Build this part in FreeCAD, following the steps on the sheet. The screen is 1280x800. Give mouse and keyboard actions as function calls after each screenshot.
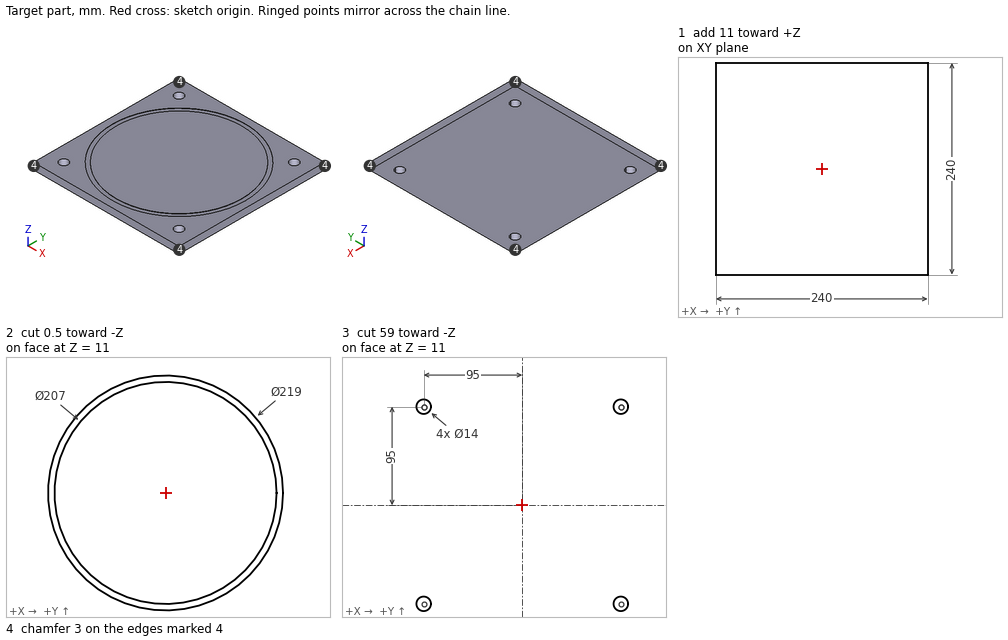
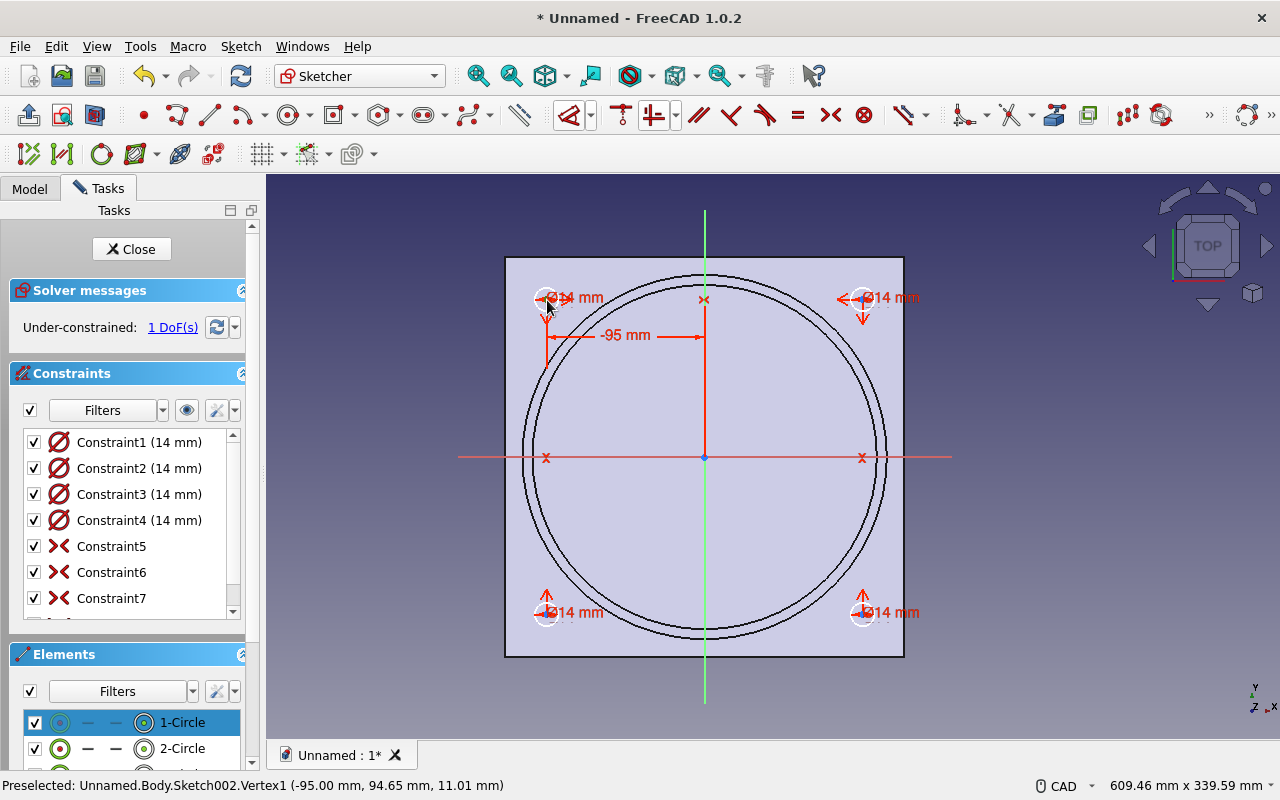
key(i)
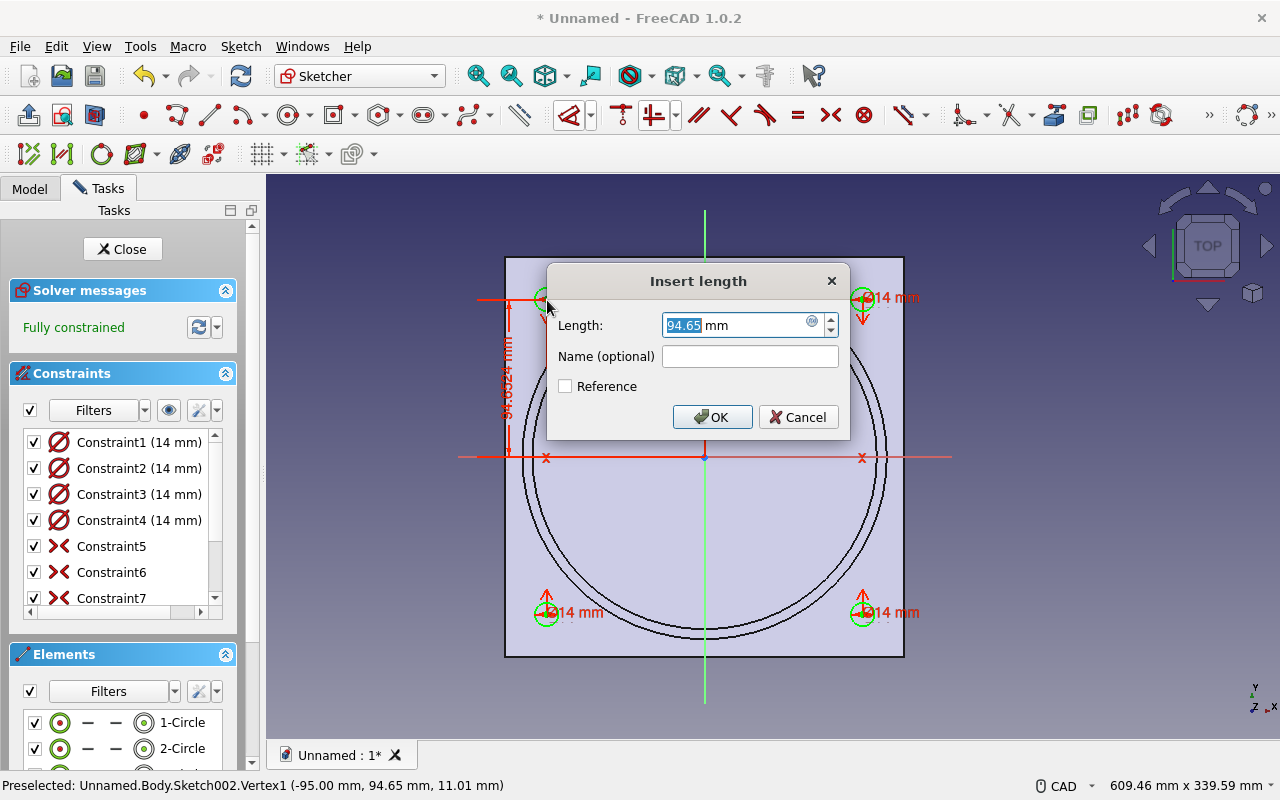
text(95)
key(Return)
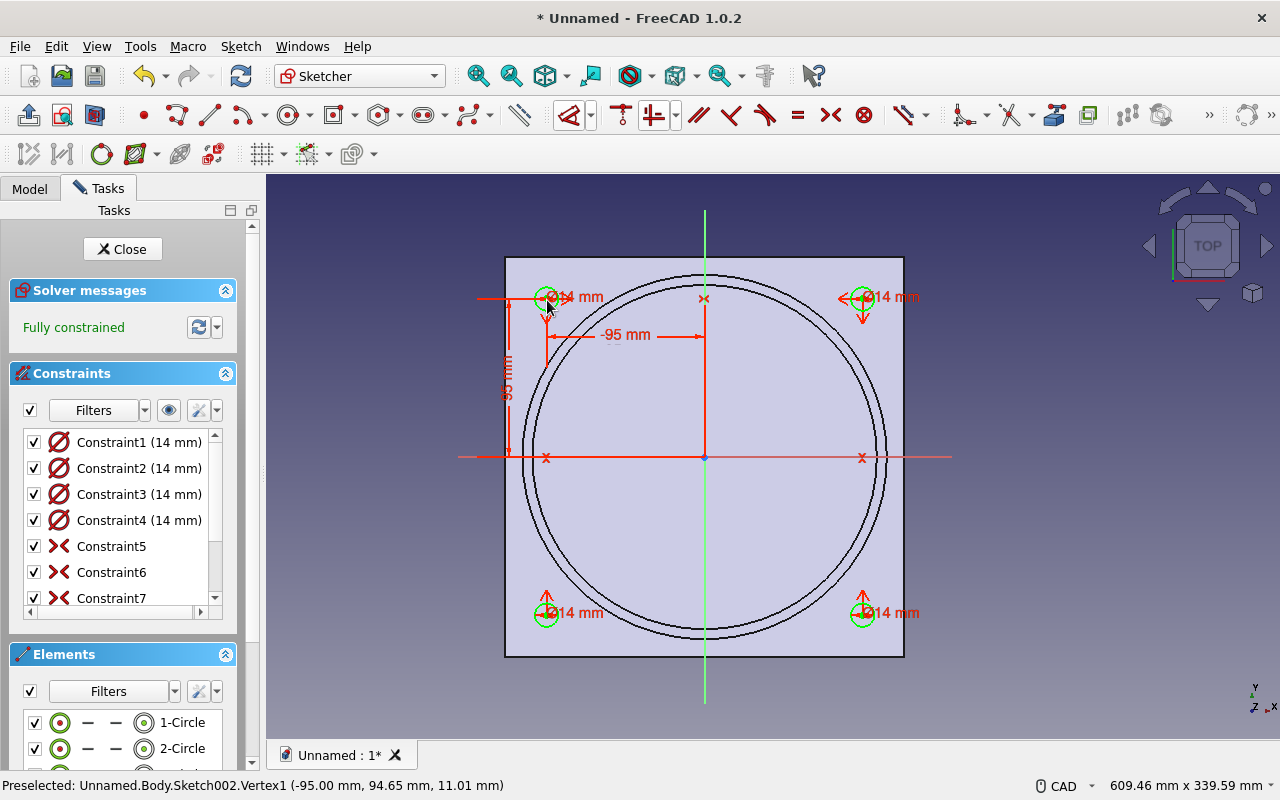
click(123, 249)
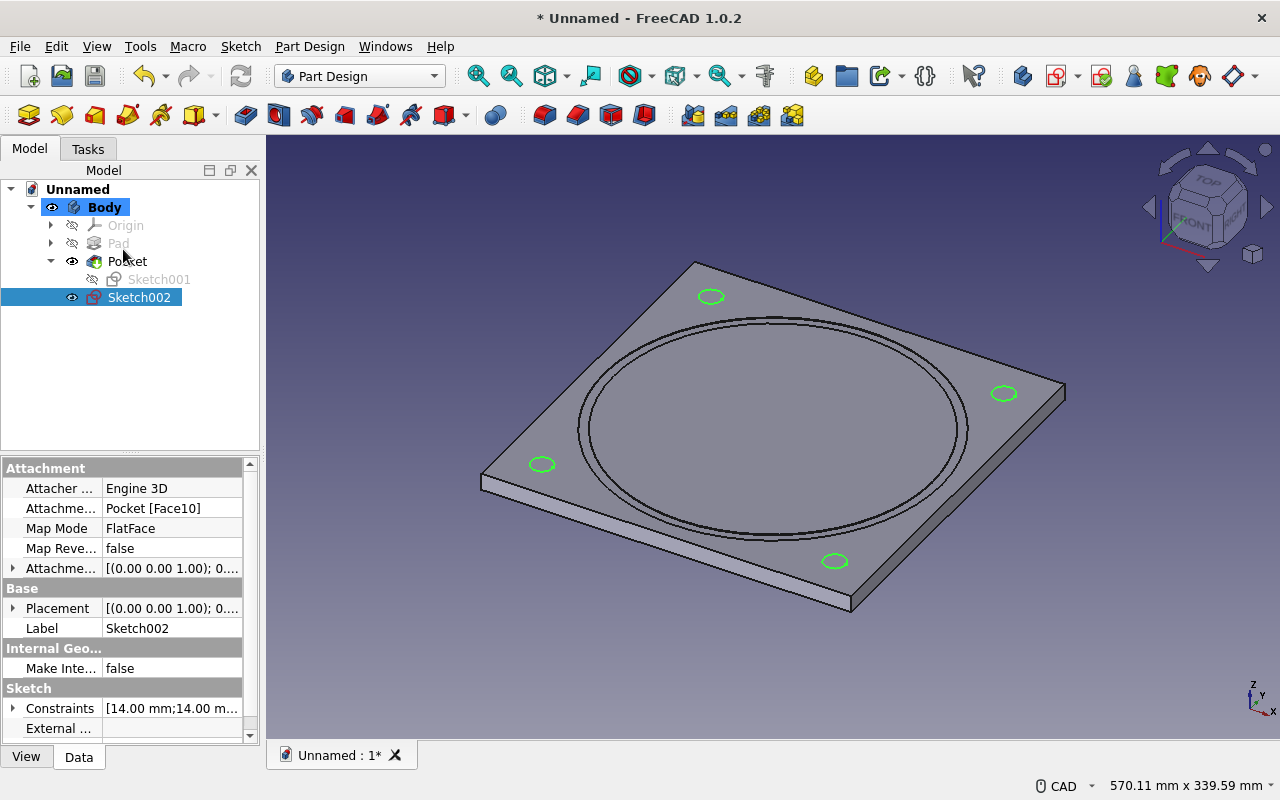
click(246, 116)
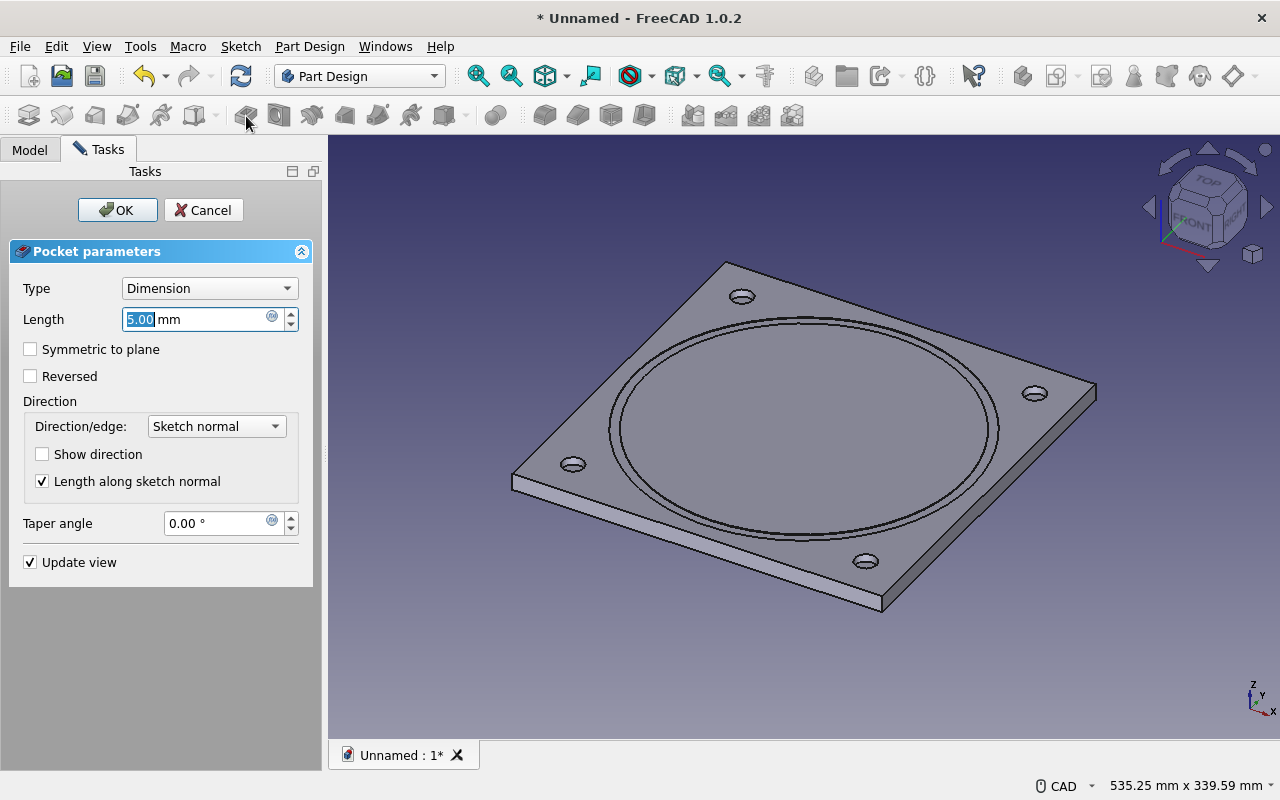
text(59)
key(Tab)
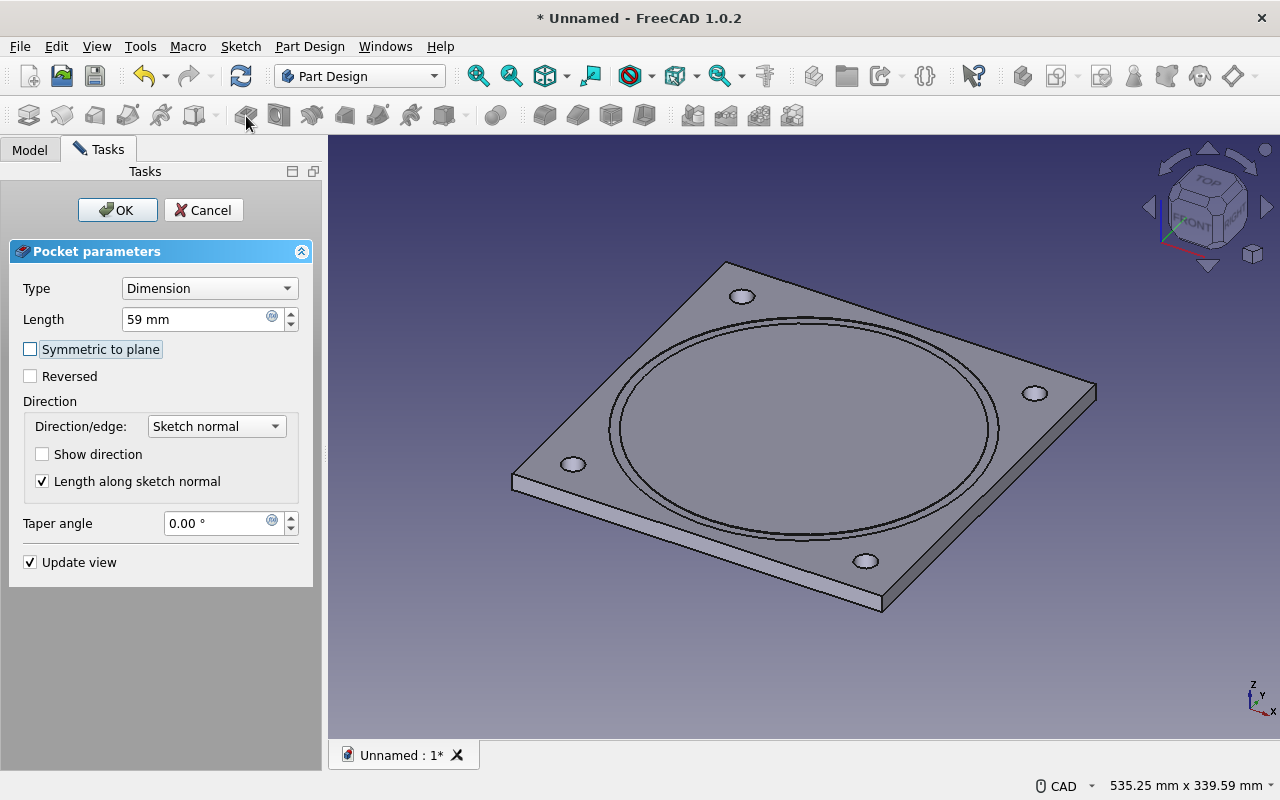
click(118, 210)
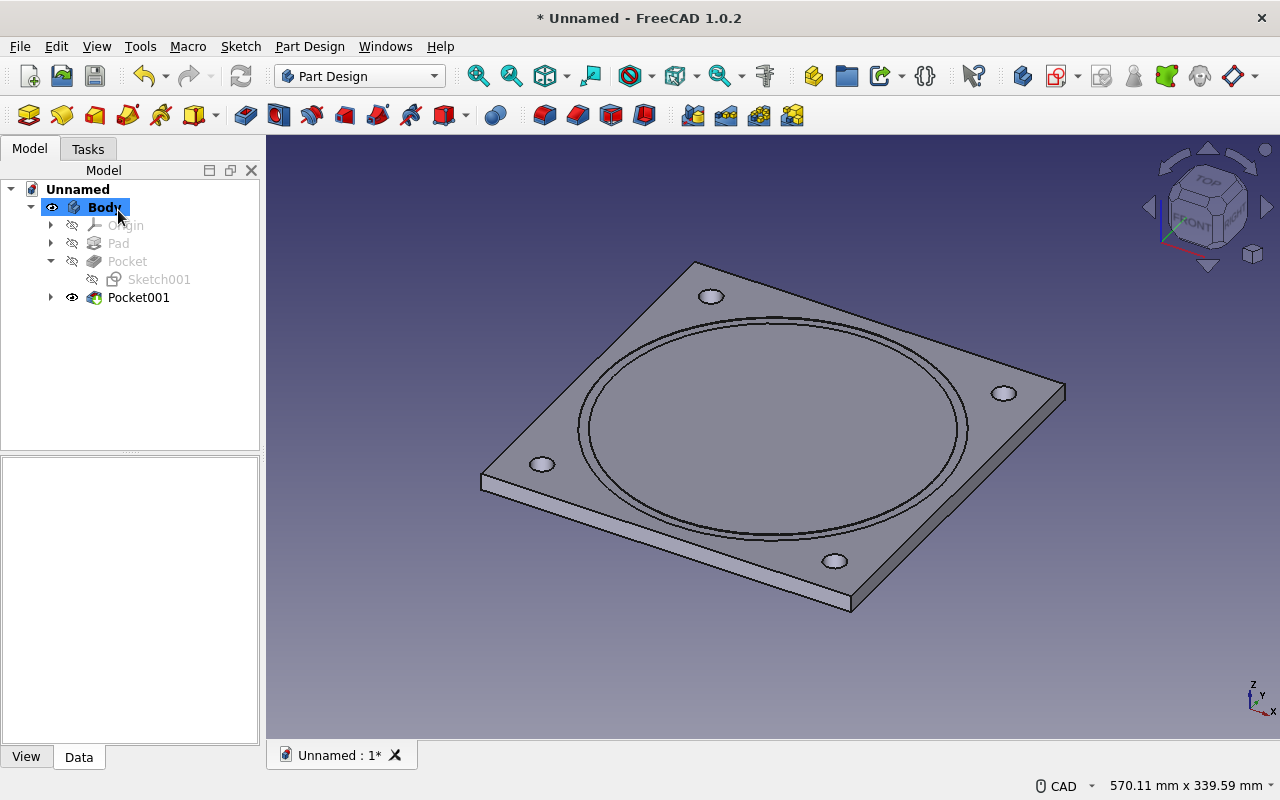
click(851, 603)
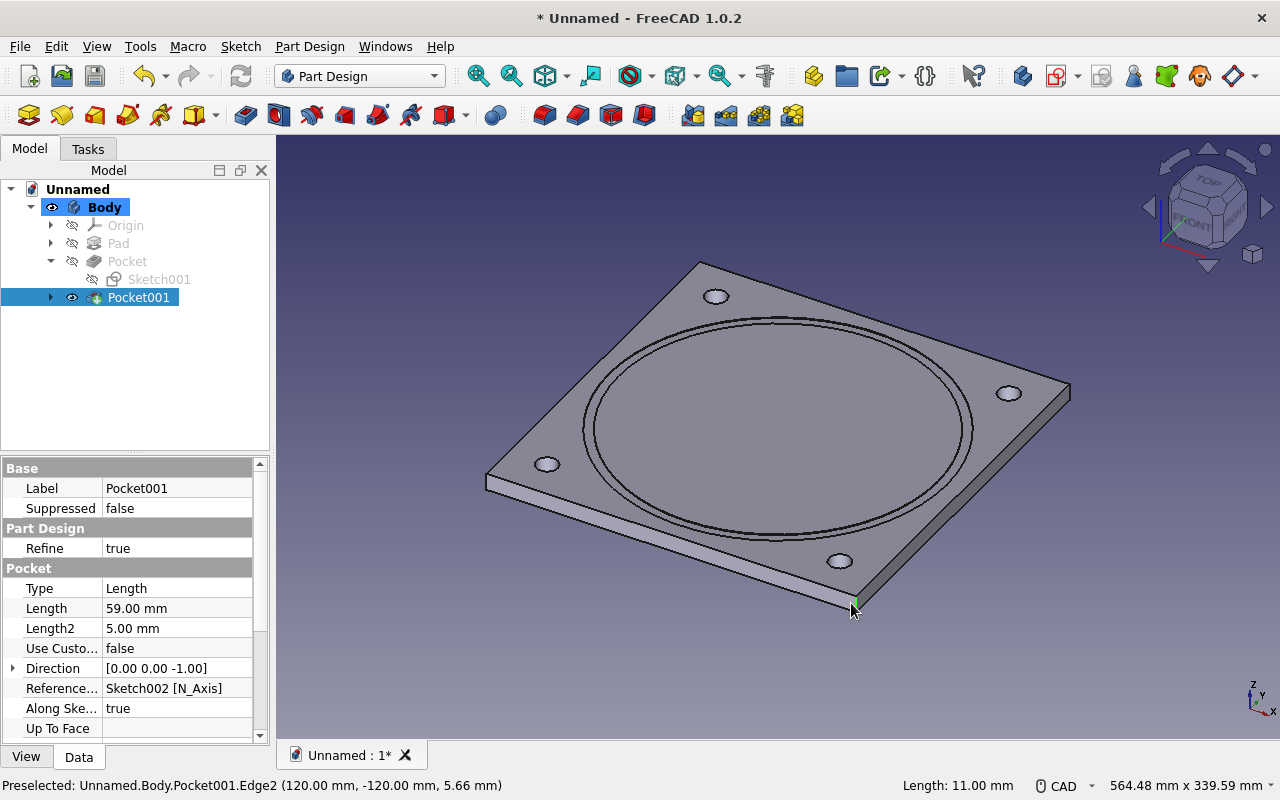
scroll(700, 269, up, 4)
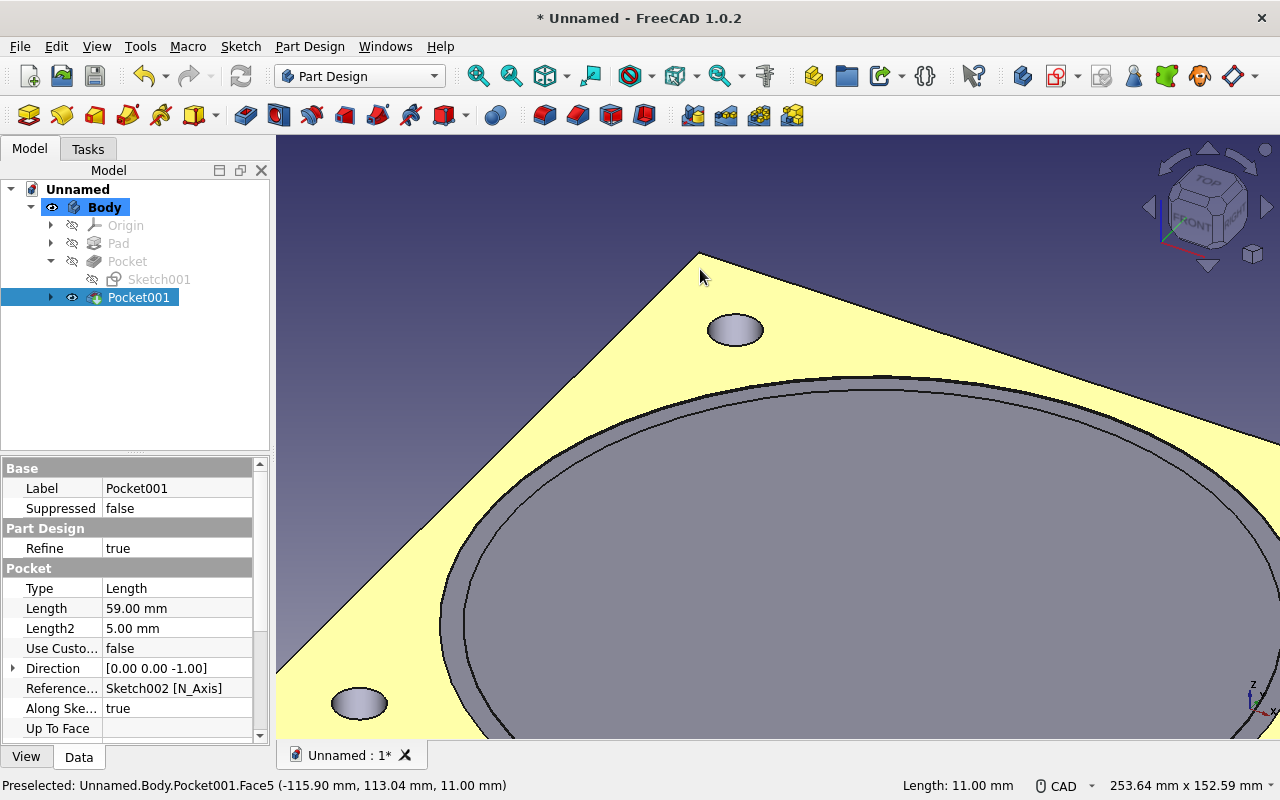
click(479, 76)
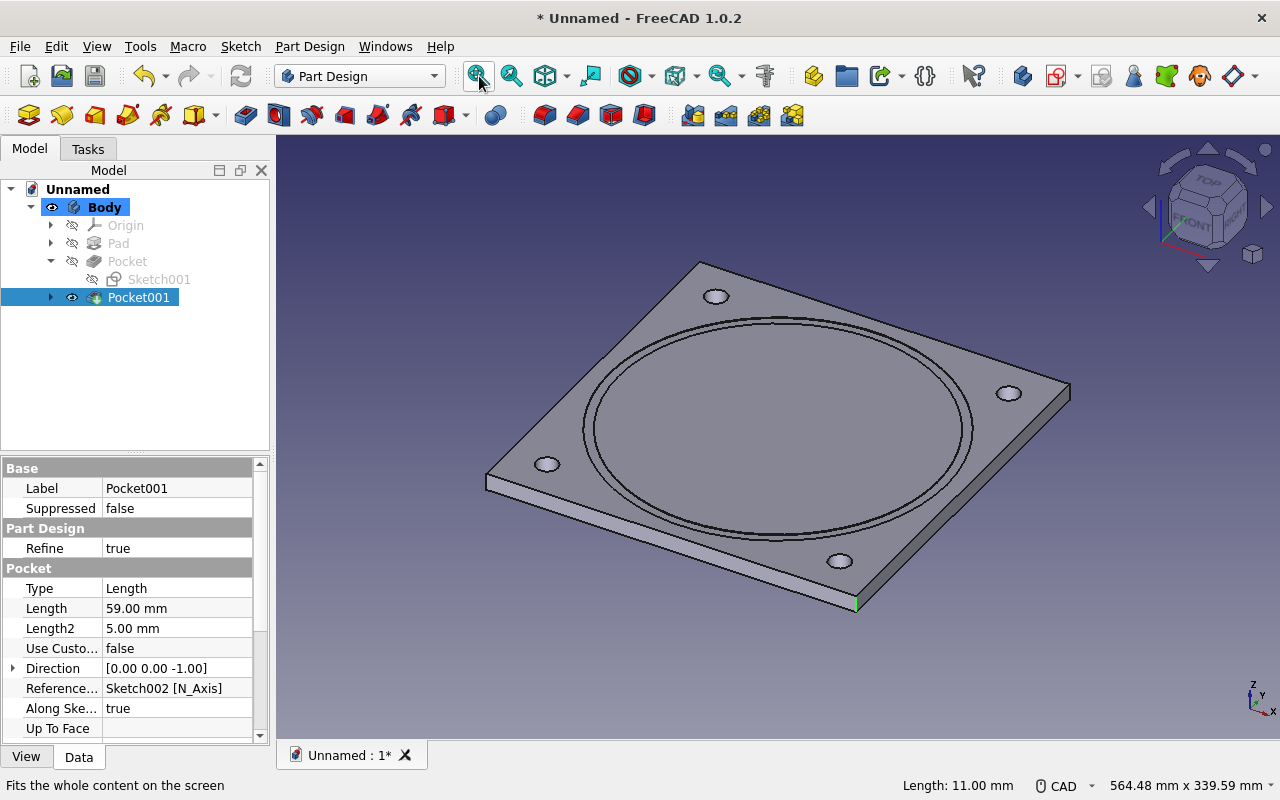
key(0)